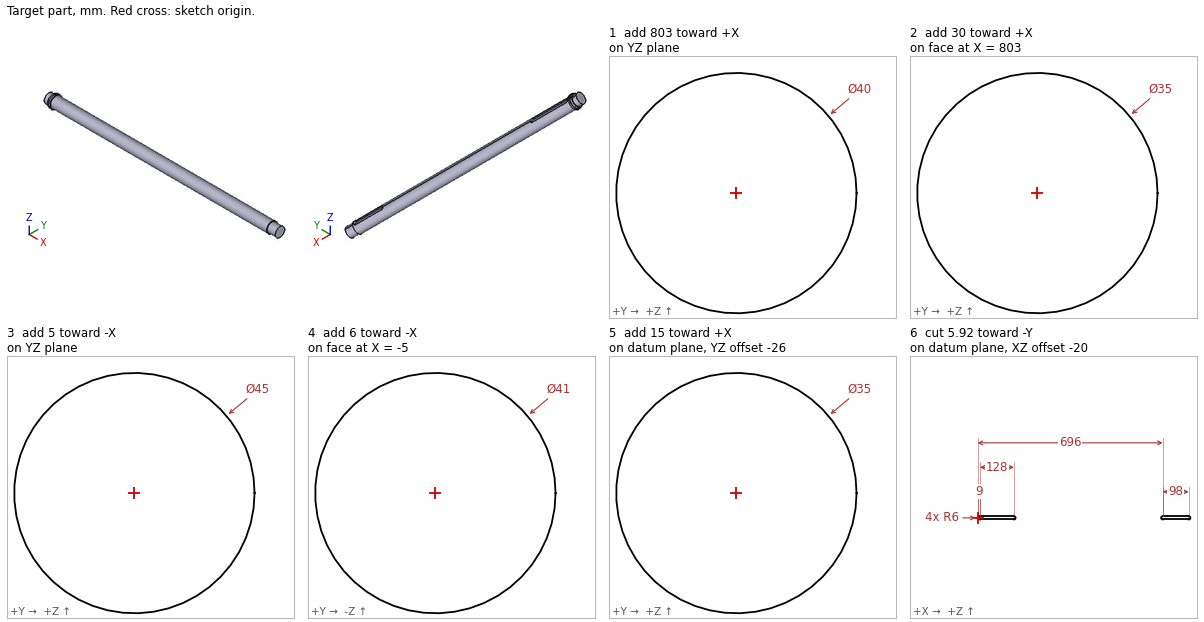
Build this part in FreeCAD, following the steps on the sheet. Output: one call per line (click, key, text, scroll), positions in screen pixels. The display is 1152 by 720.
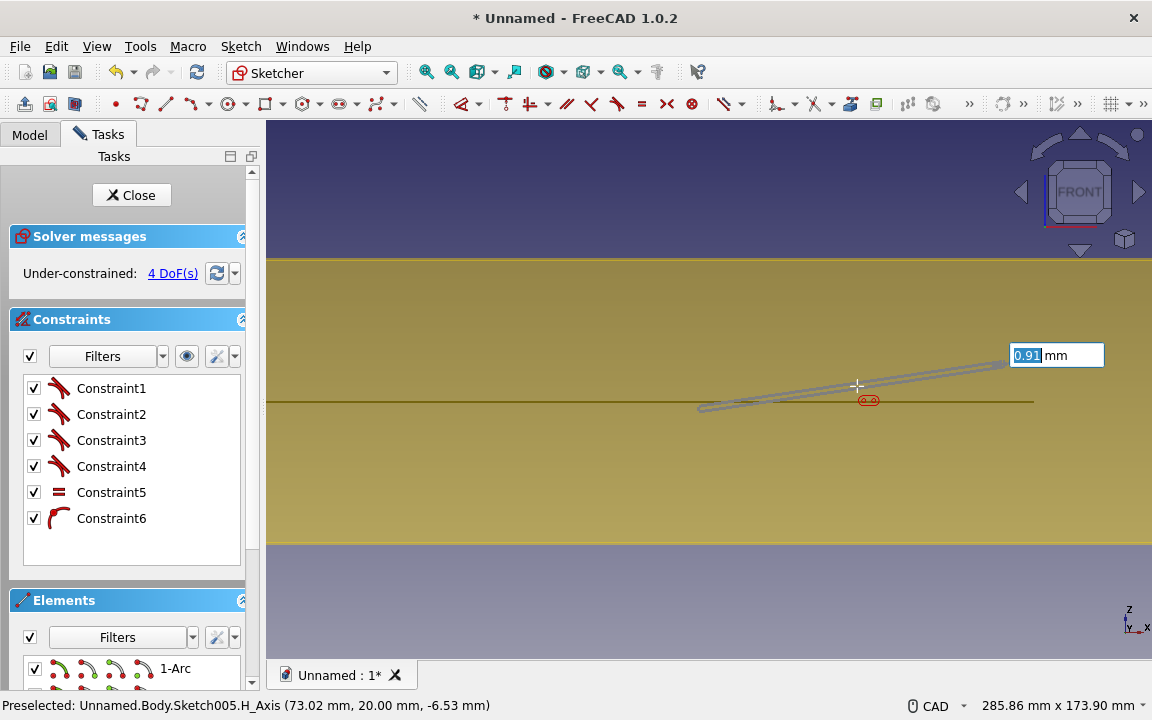
click(853, 383)
key(Escape)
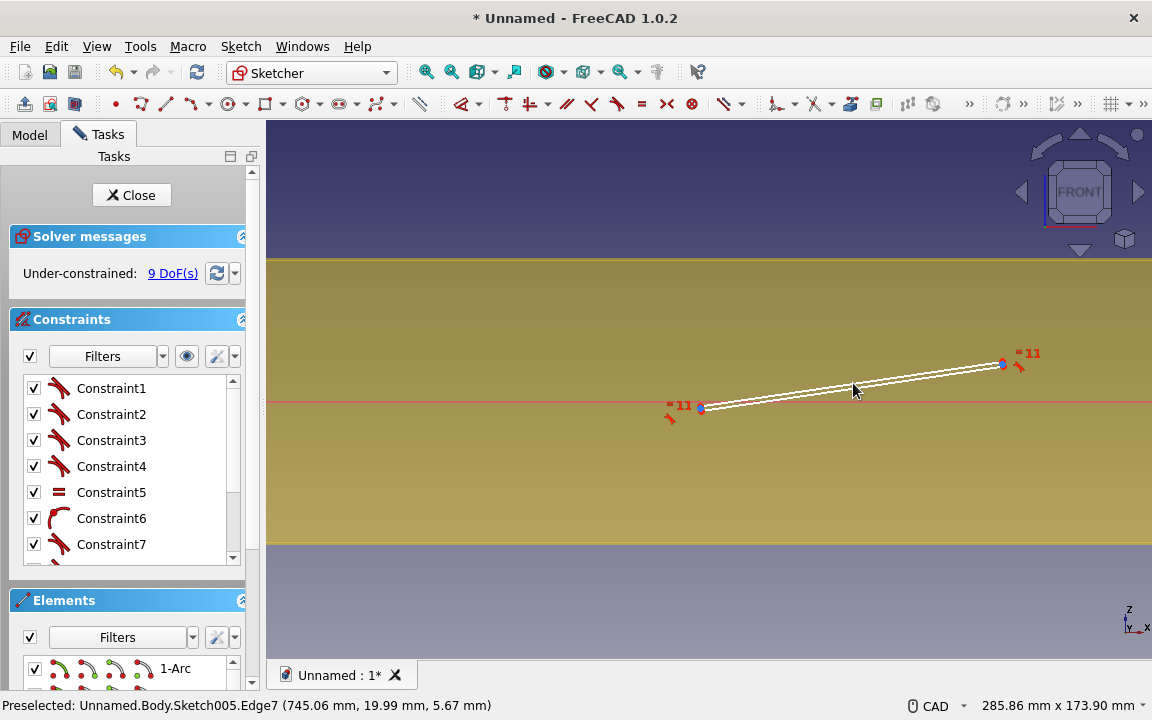
scroll(857, 386, down, 8)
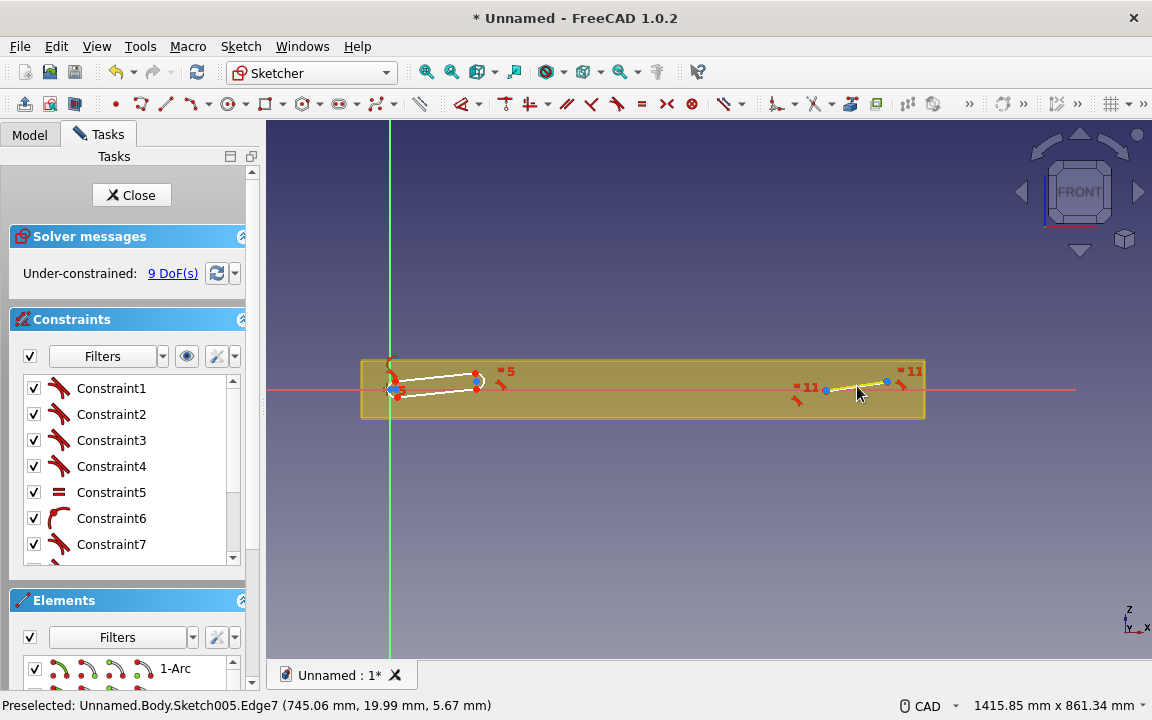
scroll(419, 379, up, 2)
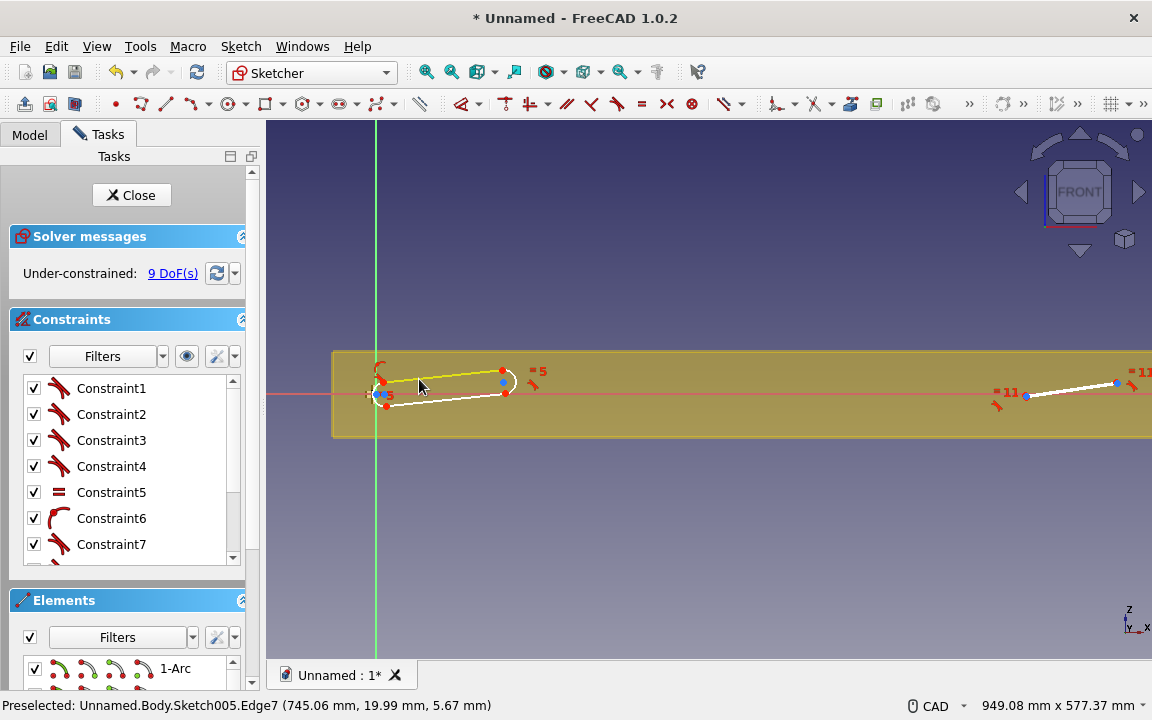
click(419, 379)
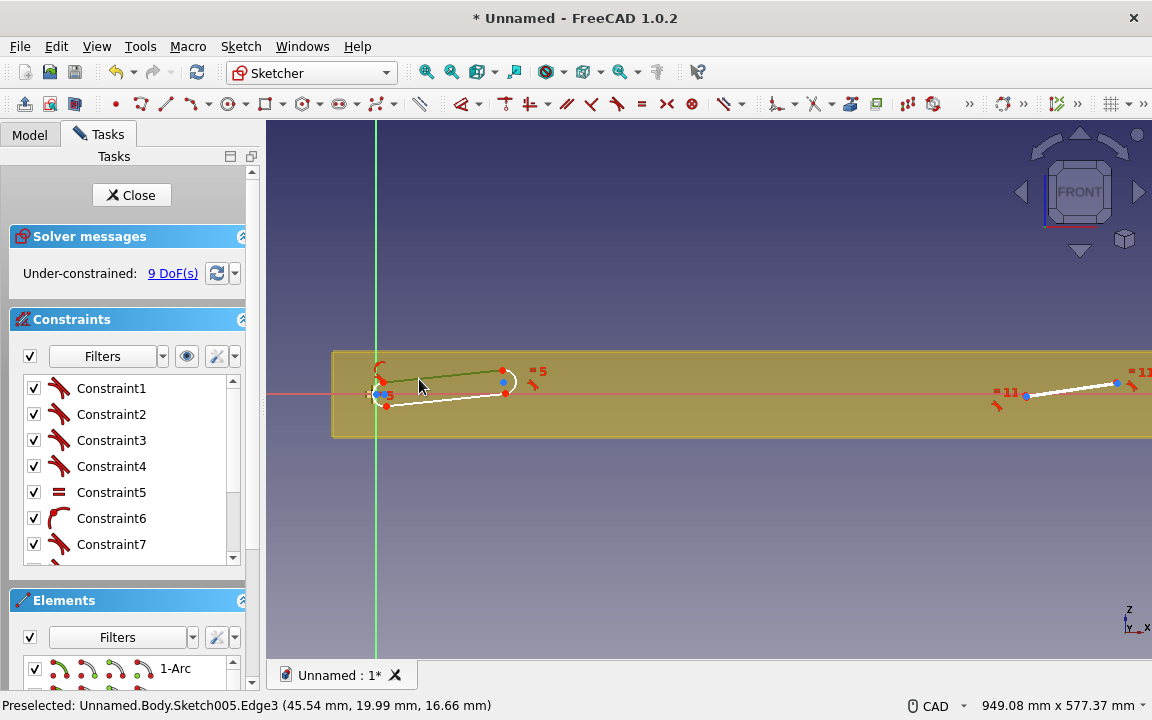
click(548, 104)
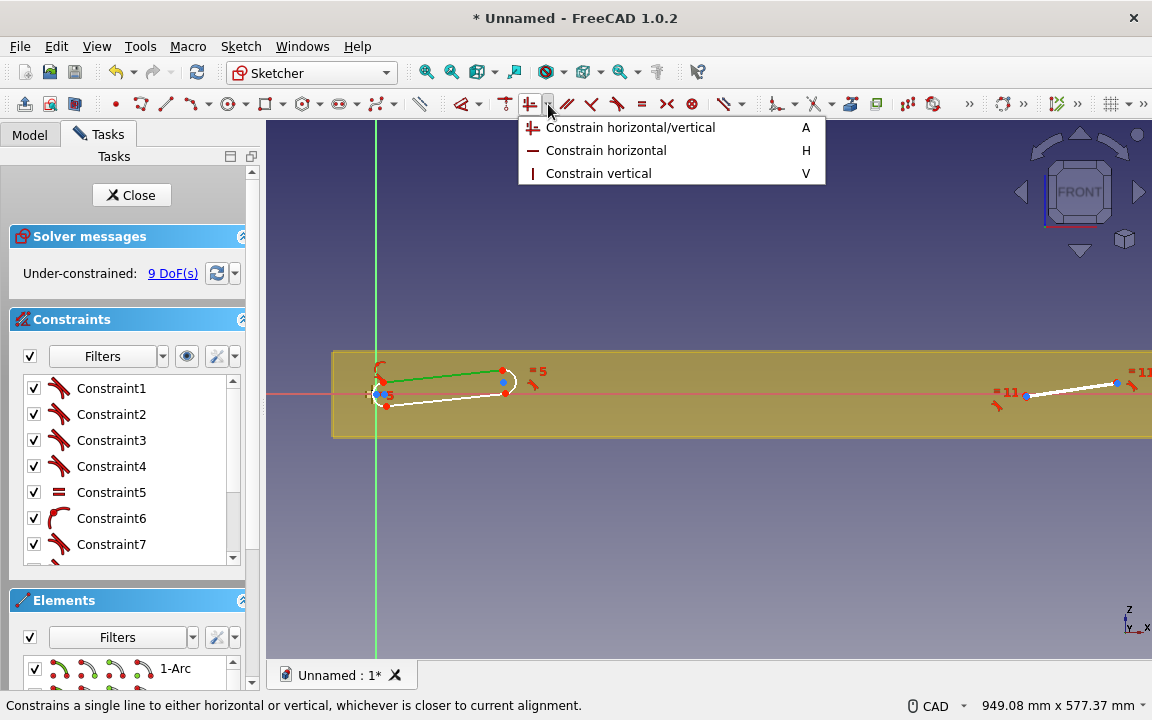
click(672, 150)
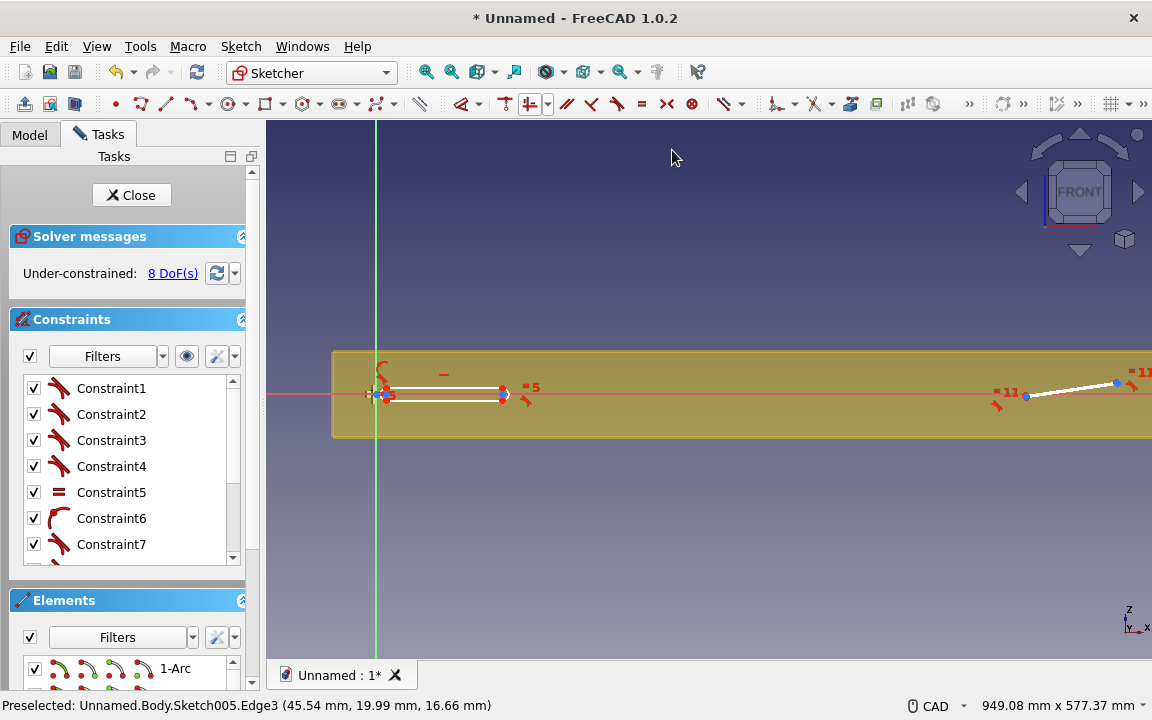
scroll(418, 379, down, 2)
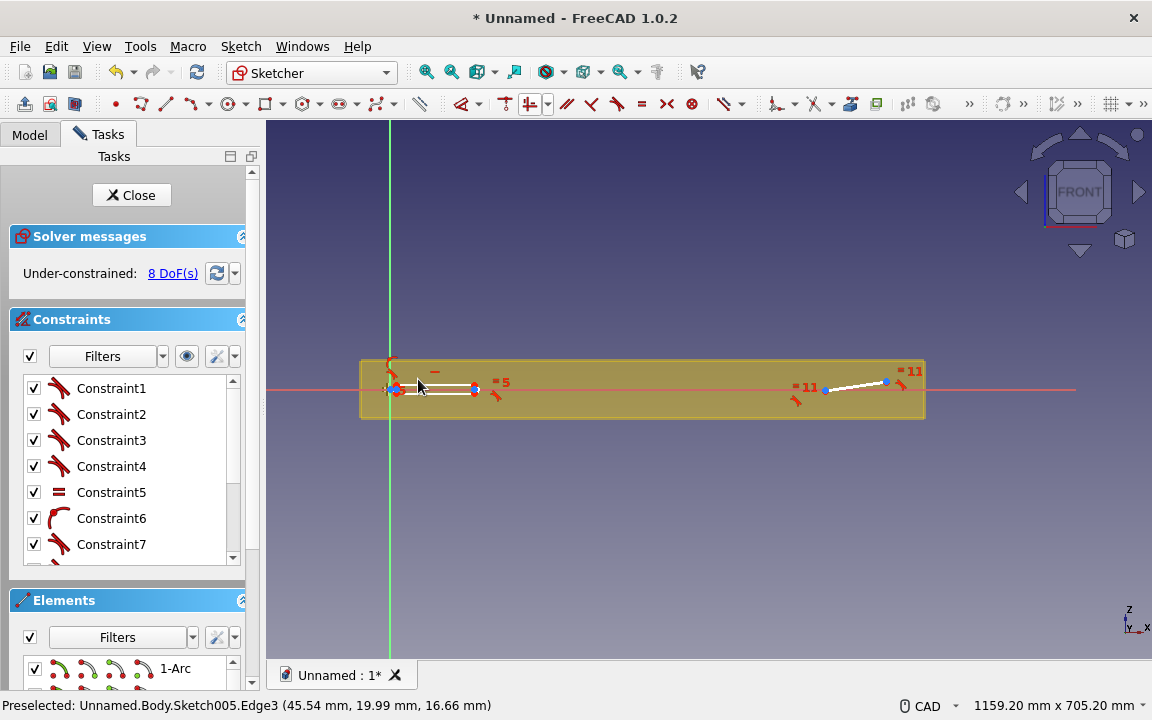
scroll(838, 389, up, 14)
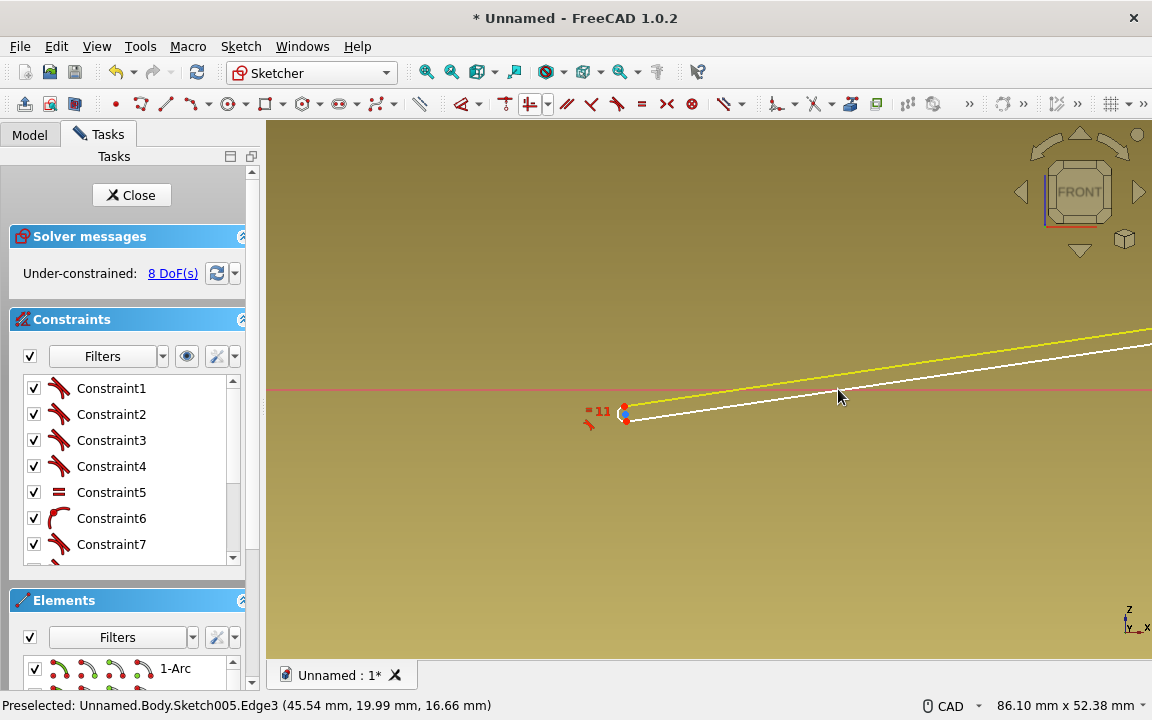
click(825, 377)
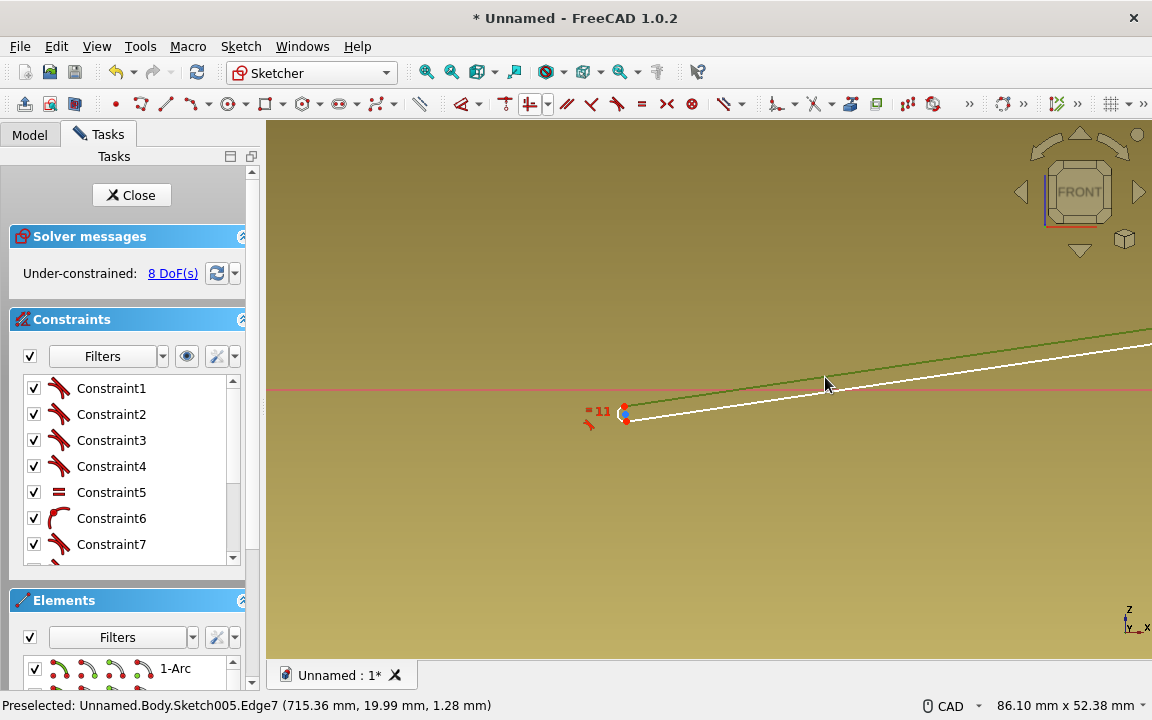
click(548, 104)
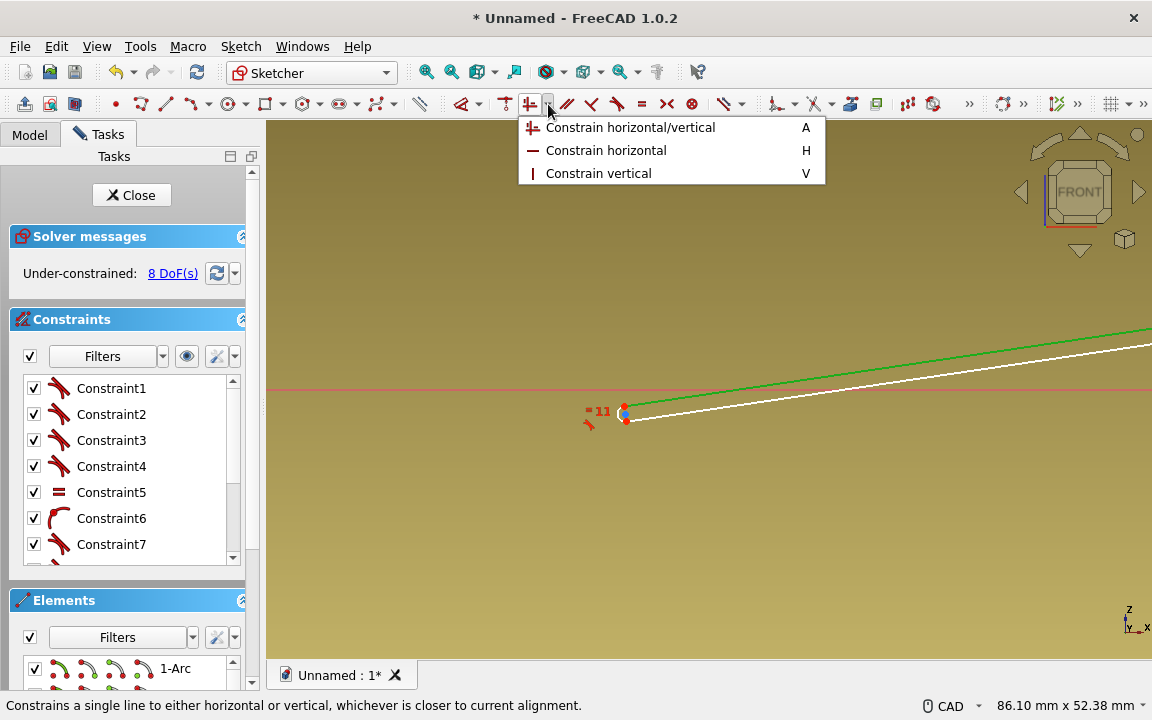
click(672, 150)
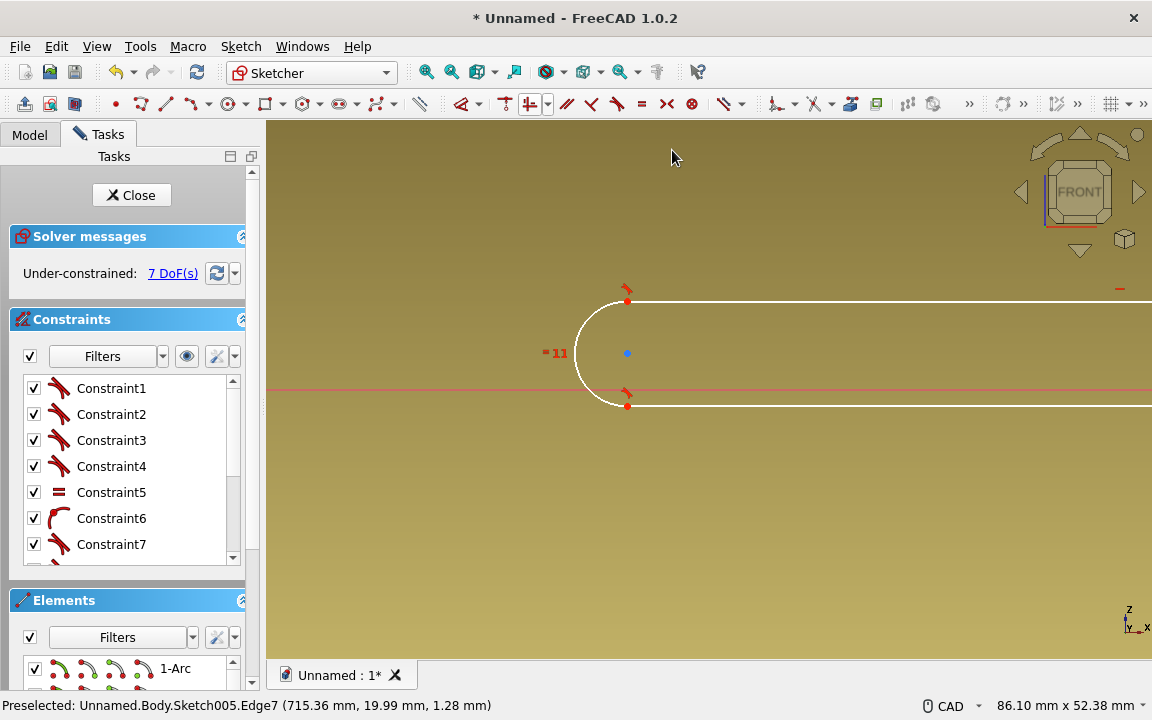
scroll(839, 389, down, 14)